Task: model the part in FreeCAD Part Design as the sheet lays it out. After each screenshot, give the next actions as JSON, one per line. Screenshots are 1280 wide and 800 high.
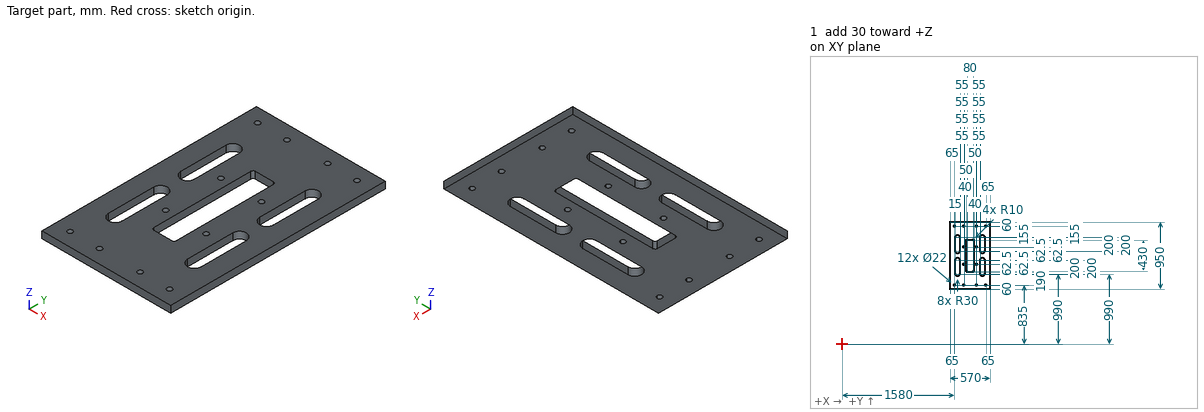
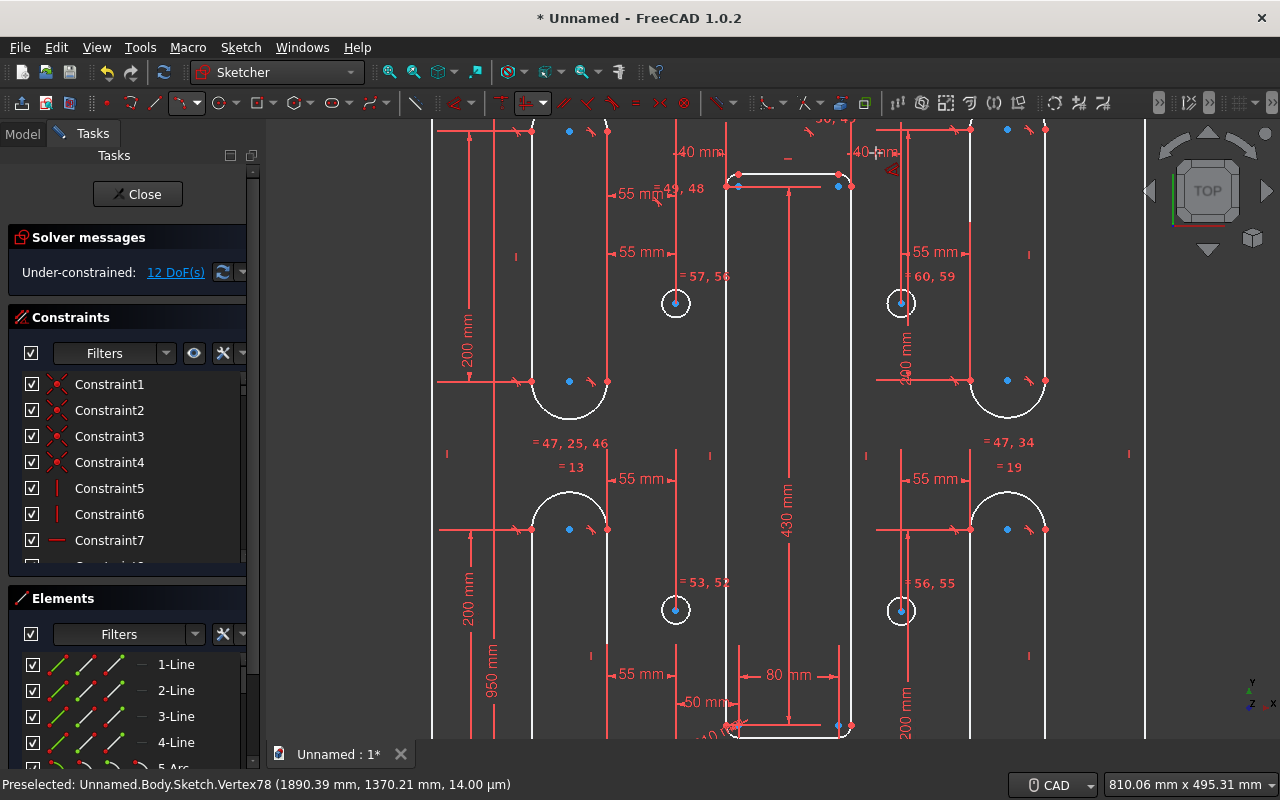
{"action": "scroll", "coordinate": [923, 300], "scroll_direction": "down", "scroll_amount": 8}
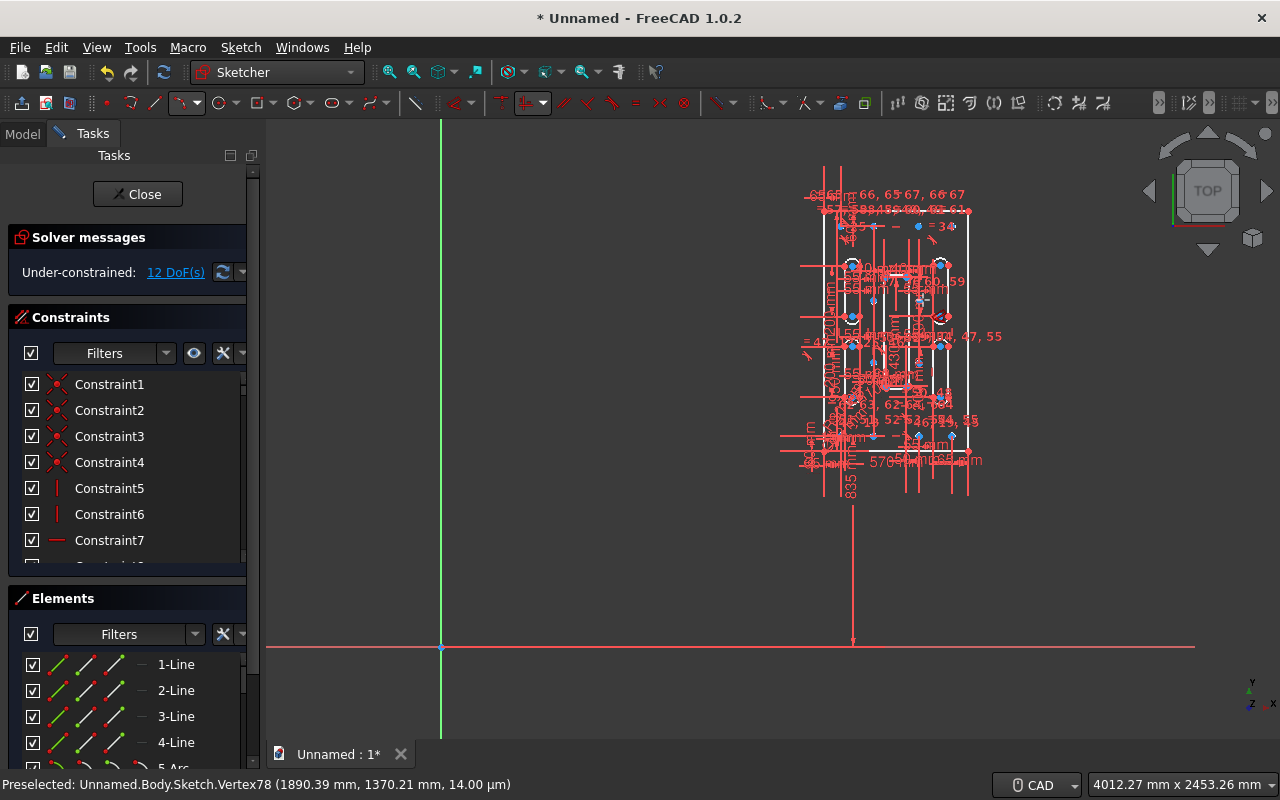
{"action": "scroll", "coordinate": [933, 266], "scroll_direction": "up", "scroll_amount": 6}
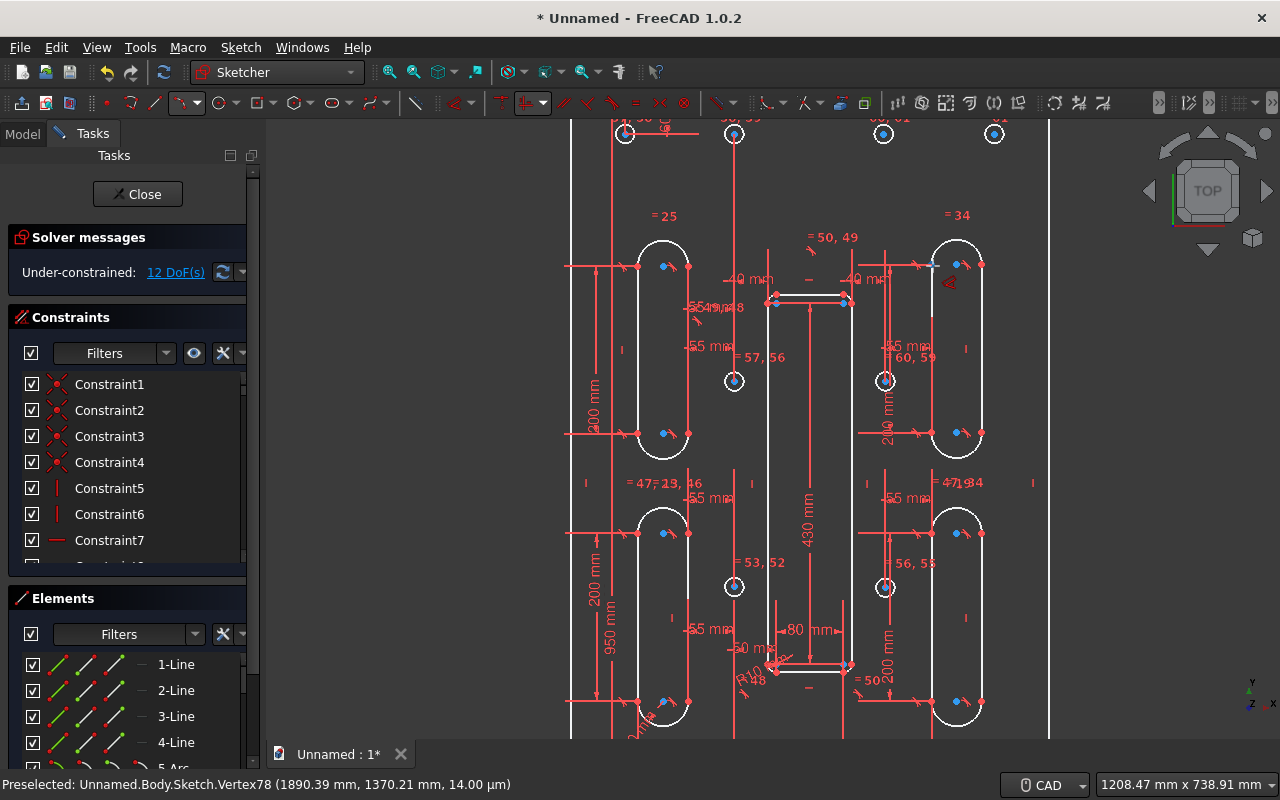
{"action": "left_click", "coordinate": [932, 265]}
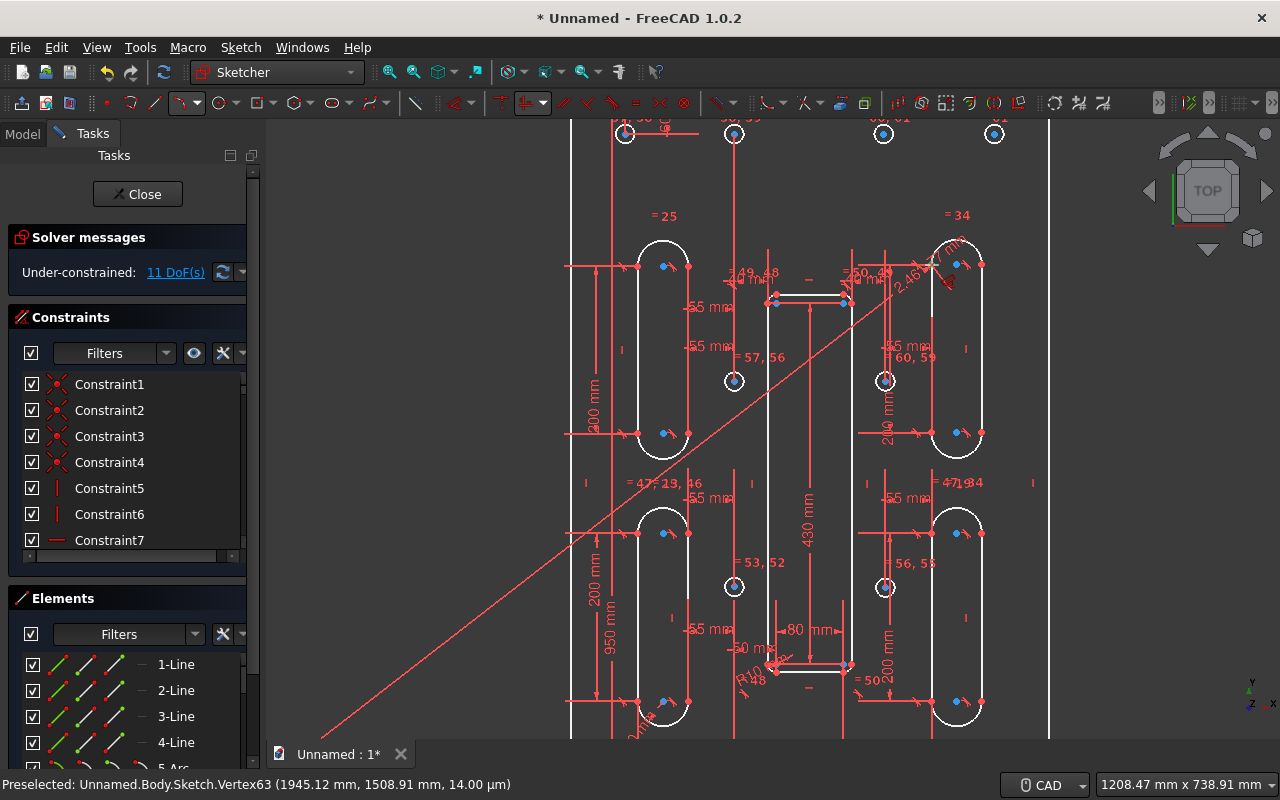
{"action": "scroll", "coordinate": [933, 266], "scroll_direction": "down", "scroll_amount": 6}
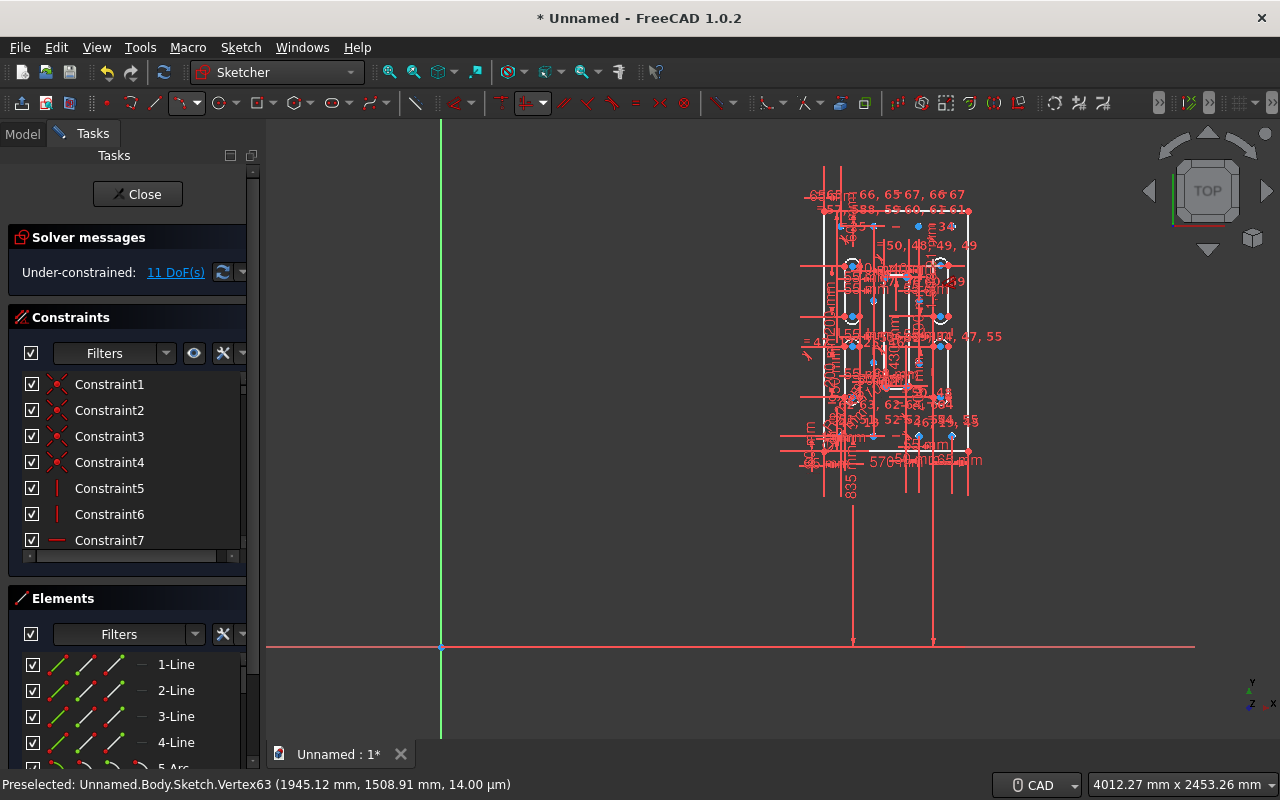
{"action": "scroll", "coordinate": [919, 226], "scroll_direction": "up", "scroll_amount": 6}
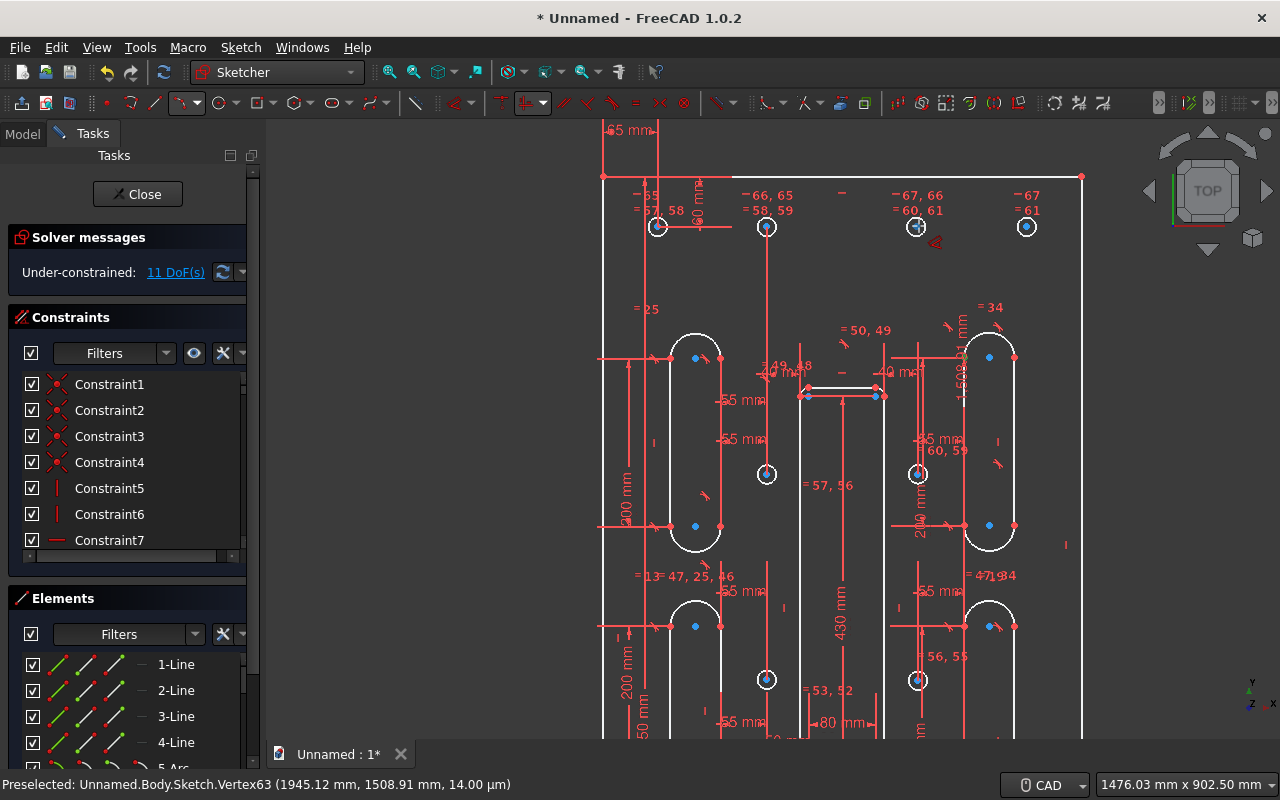
{"action": "left_click", "coordinate": [916, 227]}
{"action": "left_click", "coordinate": [940, 193]}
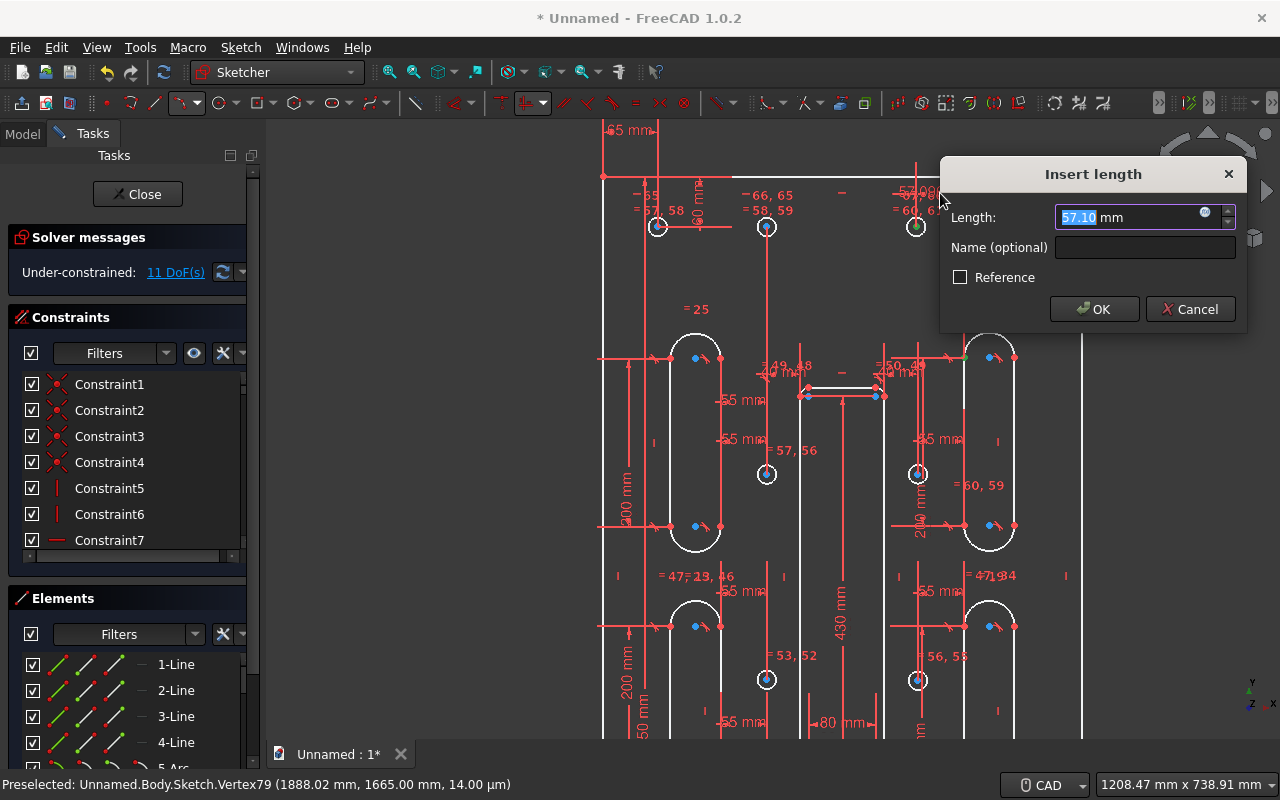
{"action": "type", "text": "55"}
{"action": "key", "text": "Return"}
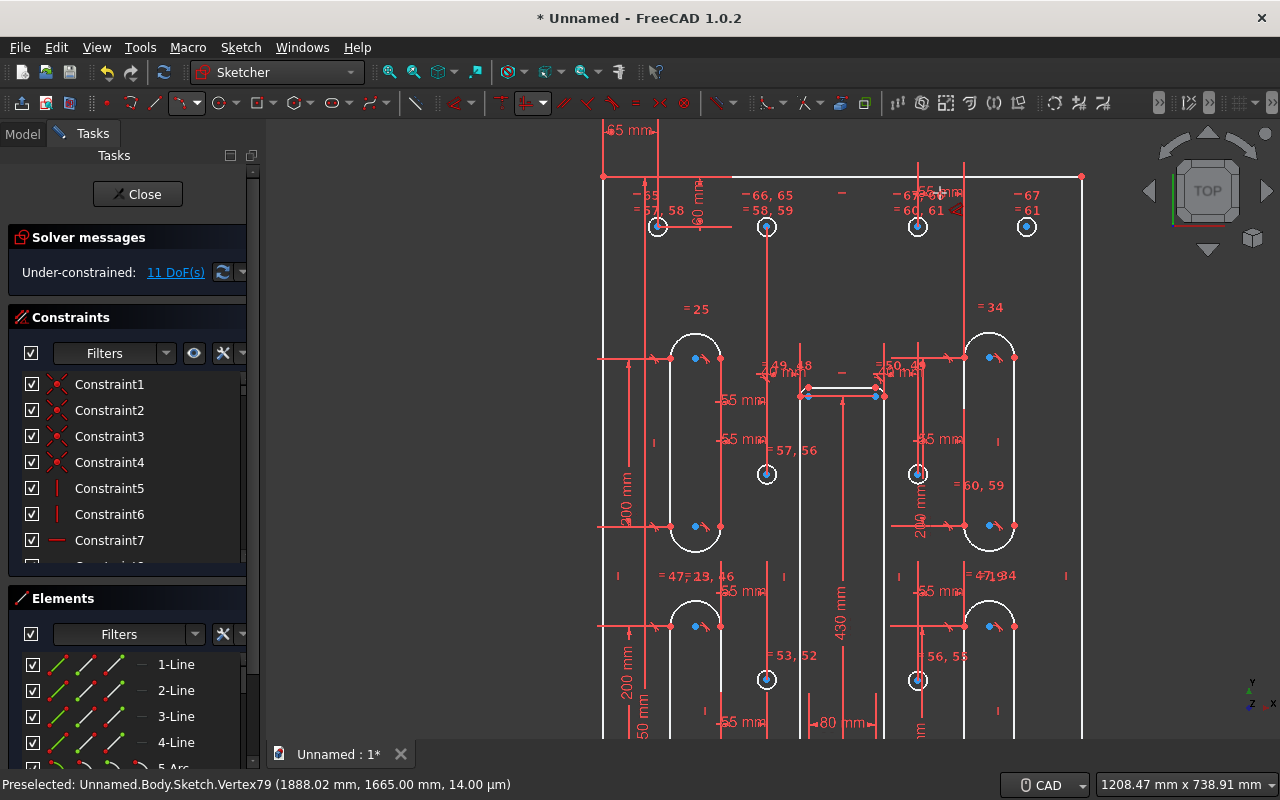
{"action": "left_click", "coordinate": [1082, 177]}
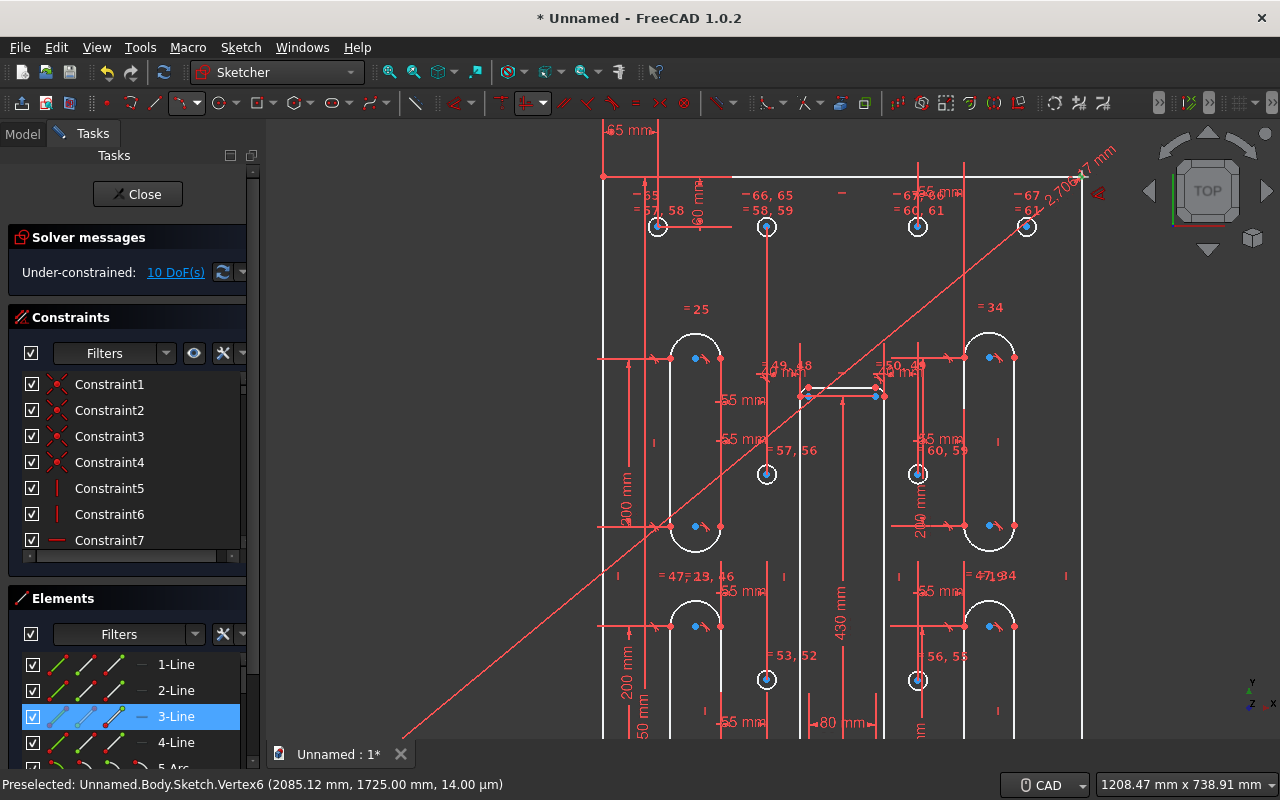
{"action": "left_click", "coordinate": [1027, 227]}
{"action": "left_click", "coordinate": [1054, 261]}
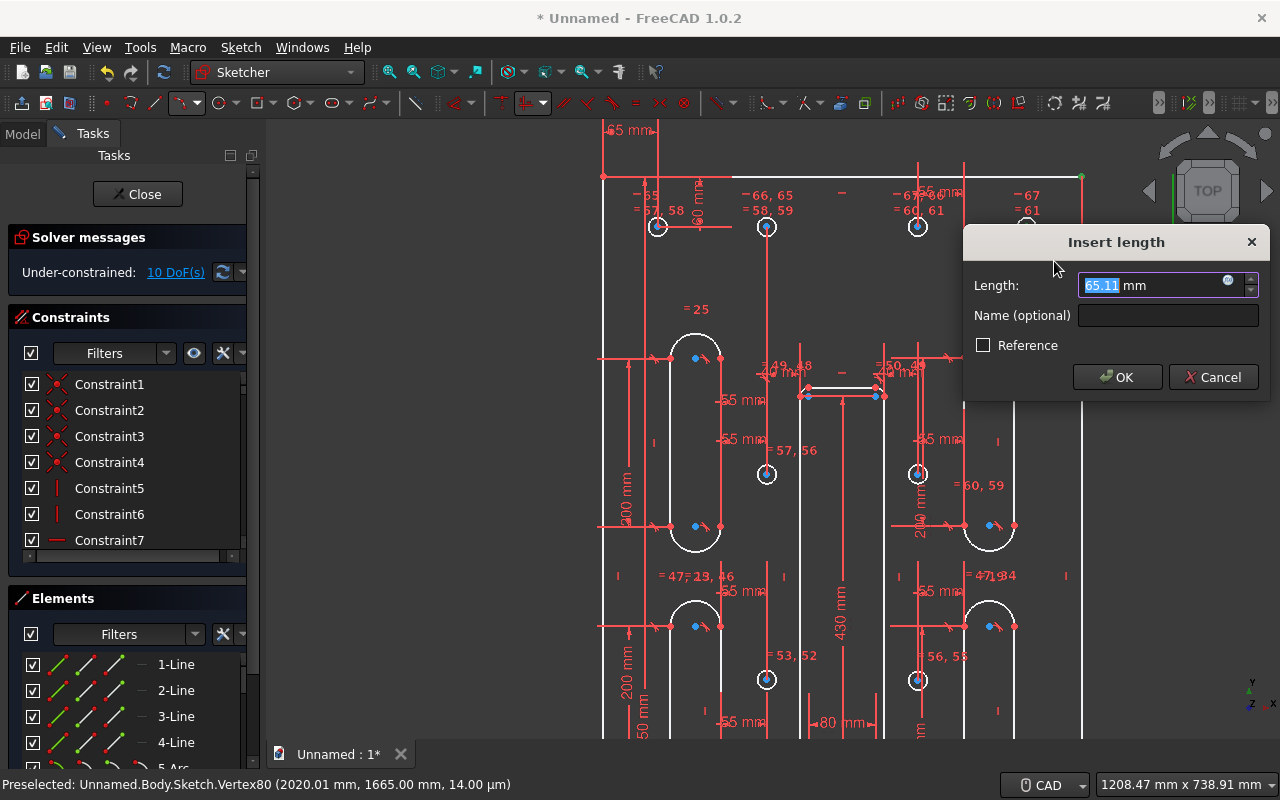
{"action": "type", "text": "65"}
{"action": "key", "text": "Return"}